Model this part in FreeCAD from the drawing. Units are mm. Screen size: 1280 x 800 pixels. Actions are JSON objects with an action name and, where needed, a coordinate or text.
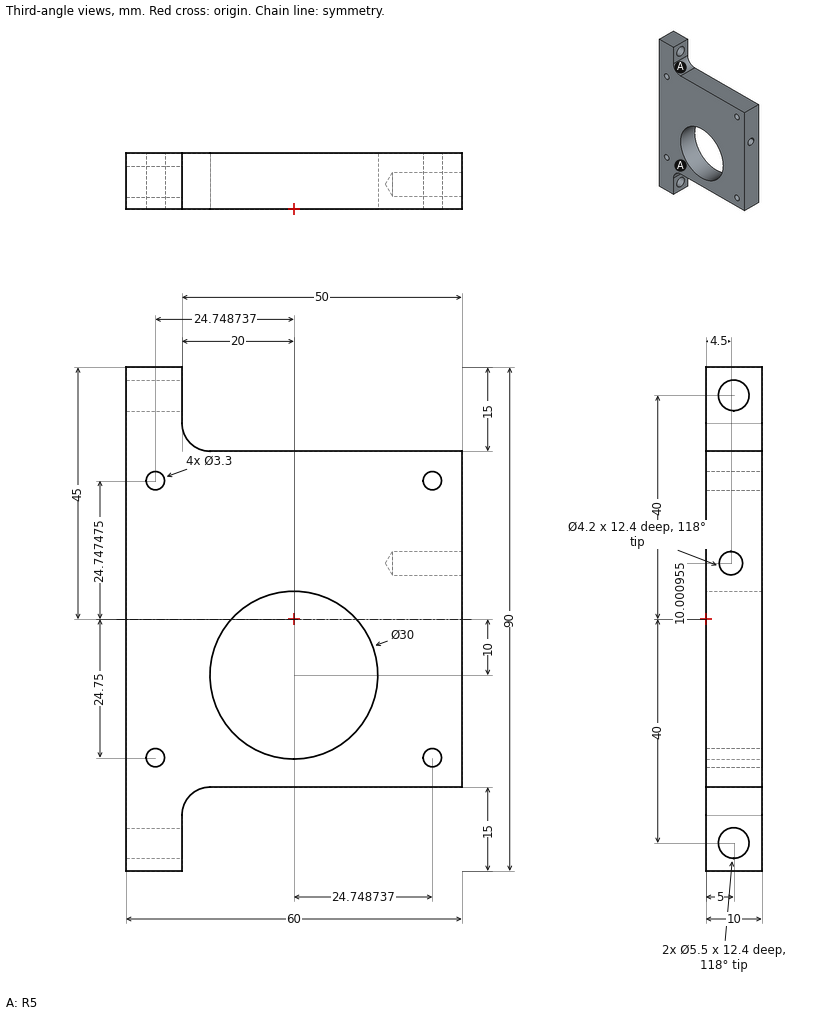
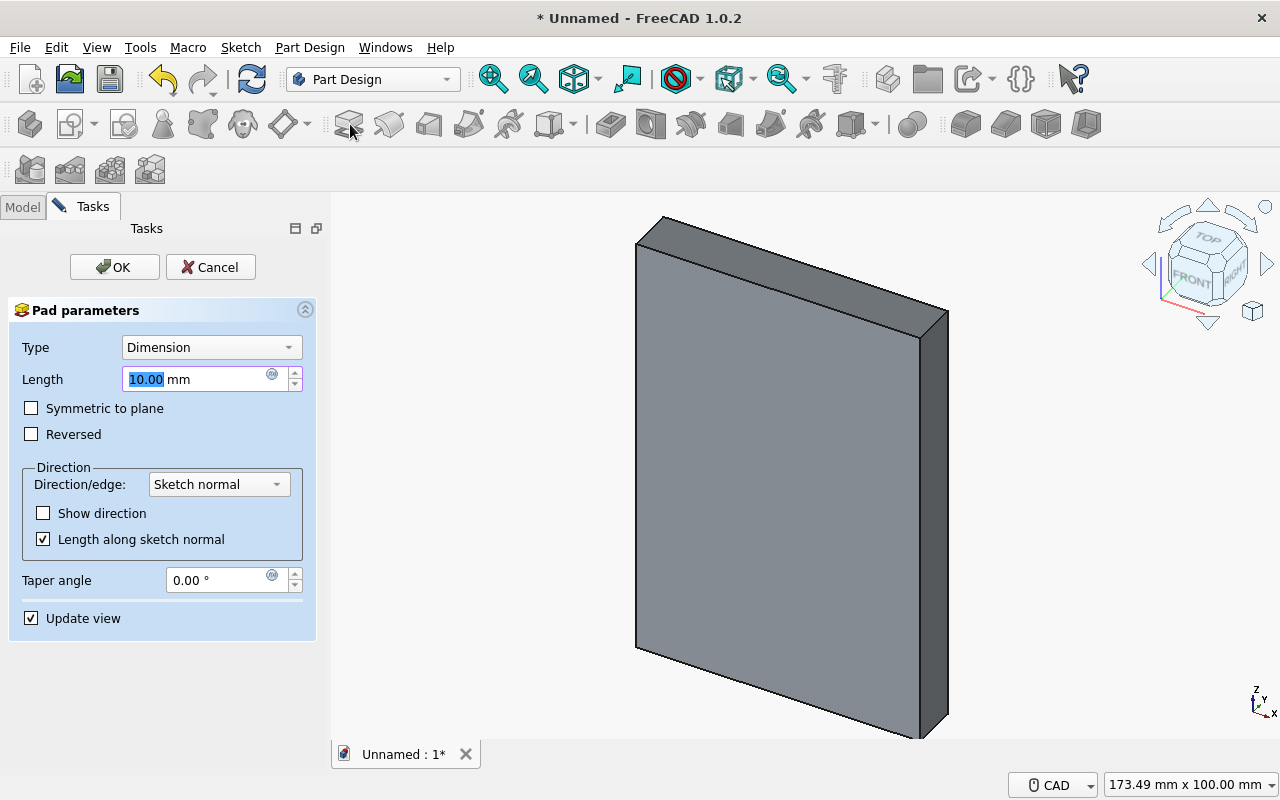
{"action": "type", "text": "10"}
{"action": "key", "text": "Tab"}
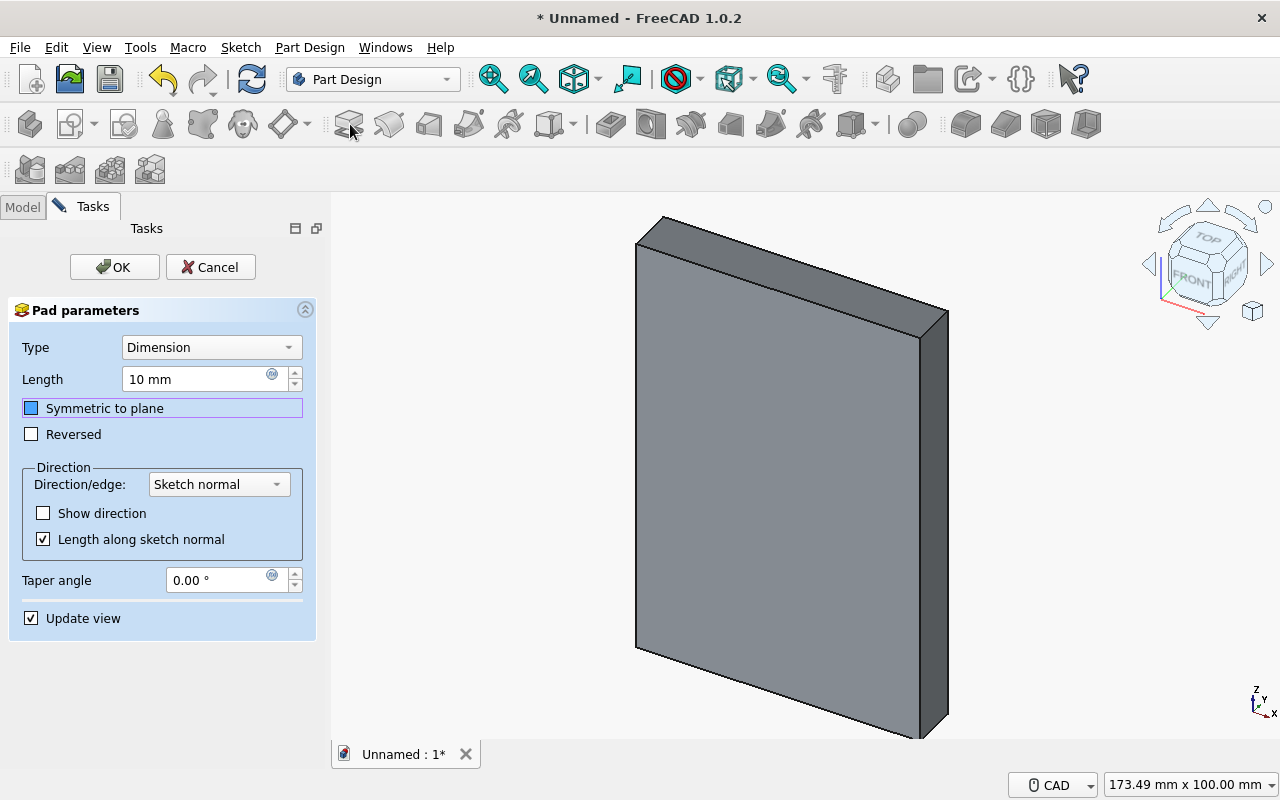
{"action": "left_click", "coordinate": [30, 434]}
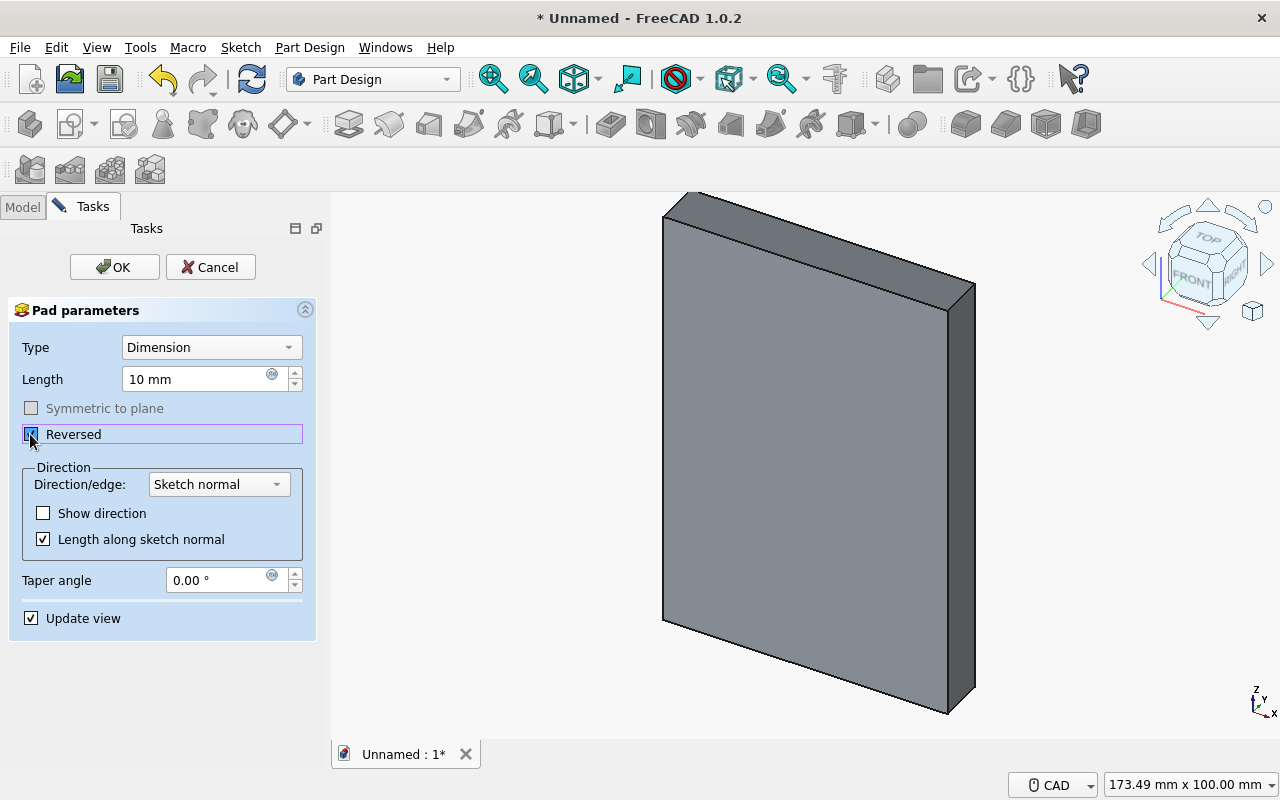
{"action": "left_click", "coordinate": [115, 267]}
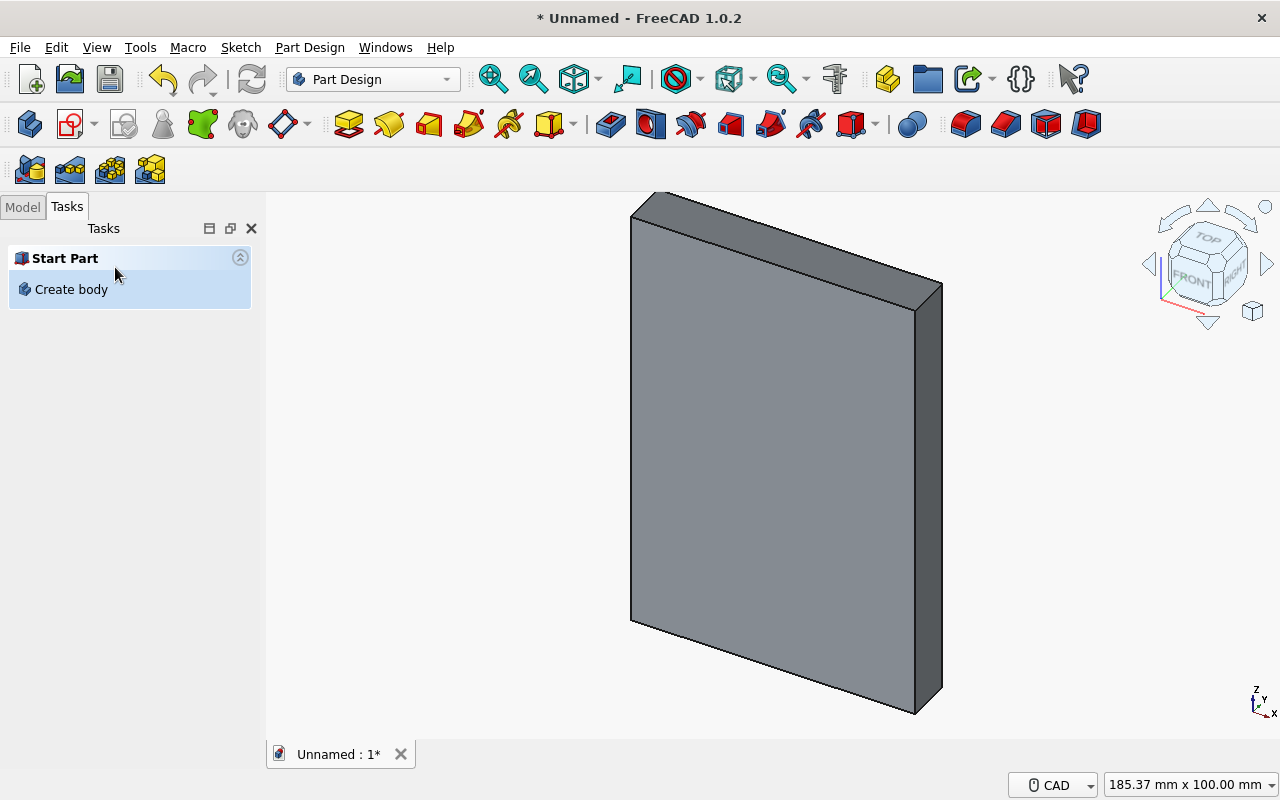
{"action": "key", "text": "v f"}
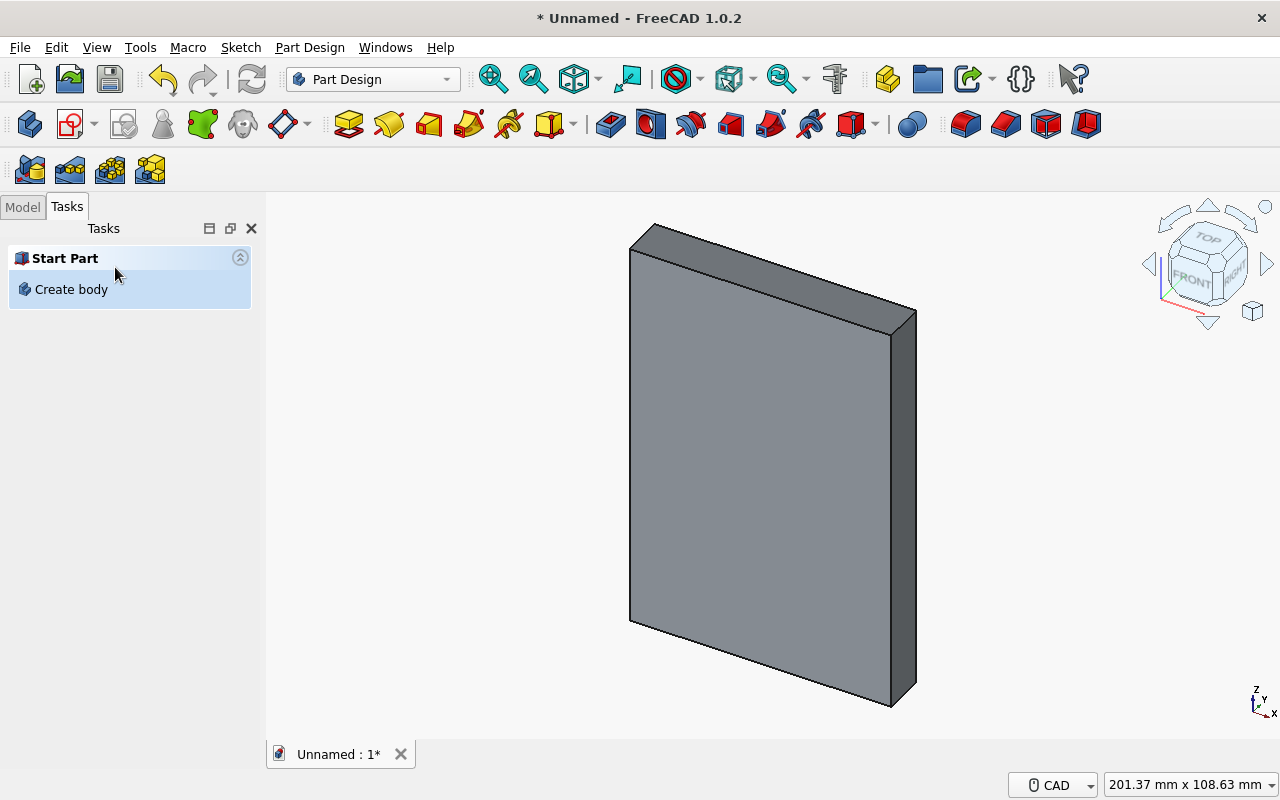
{"action": "left_click", "coordinate": [760, 424]}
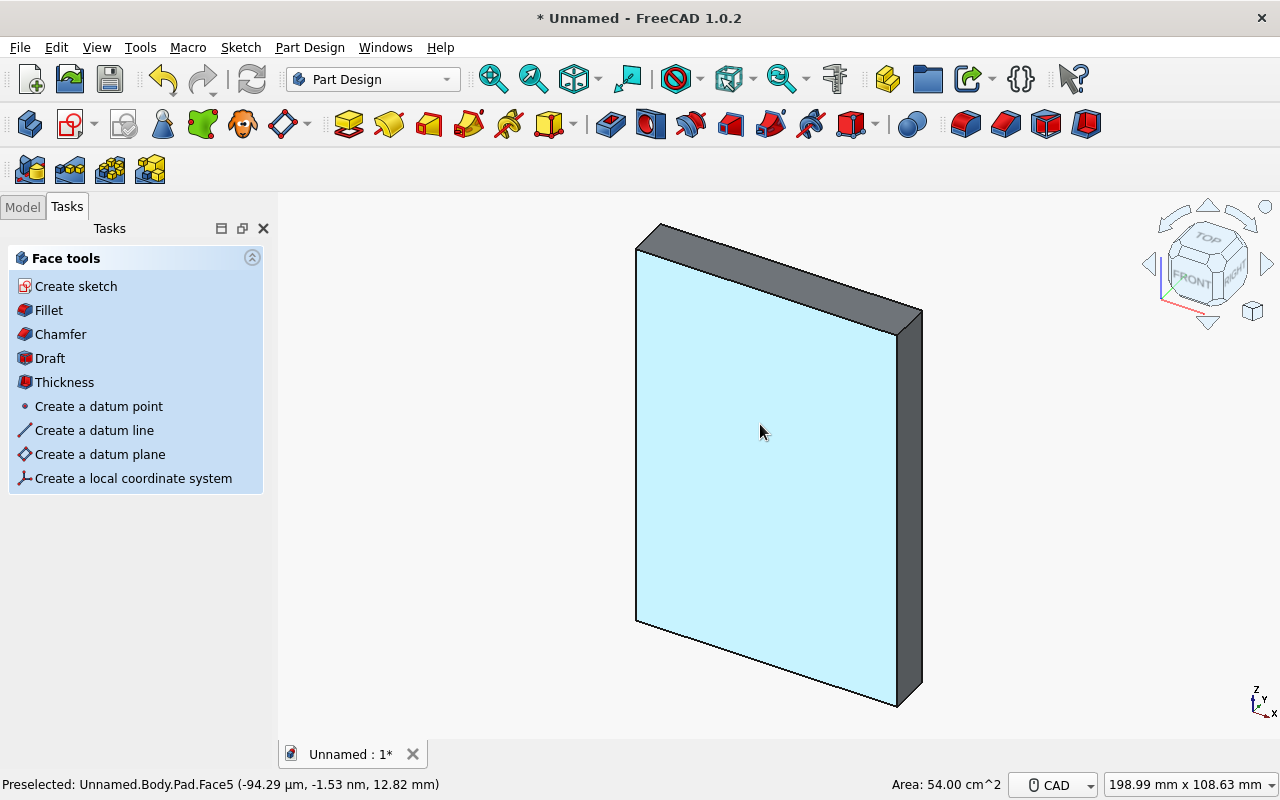
{"action": "left_click", "coordinate": [70, 124]}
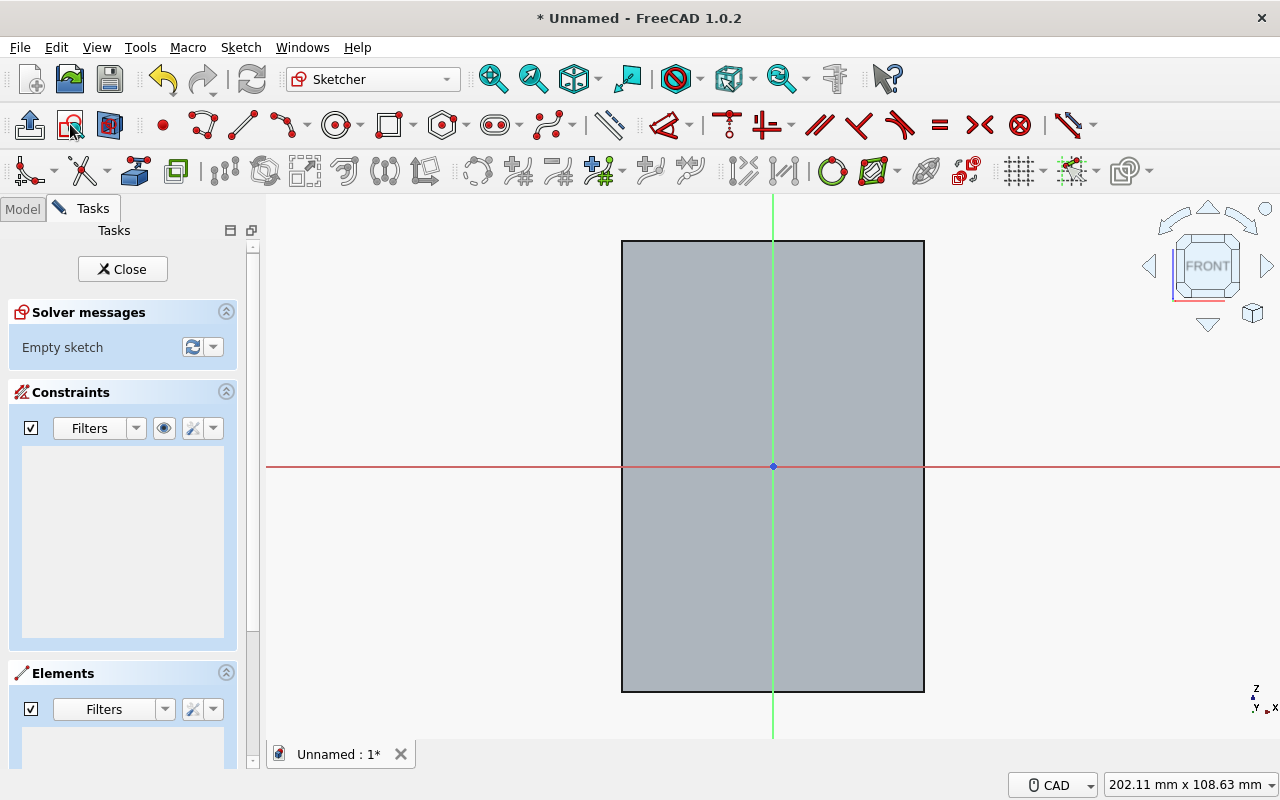
{"action": "scroll", "coordinate": [829, 558], "scroll_direction": "up", "scroll_amount": 4}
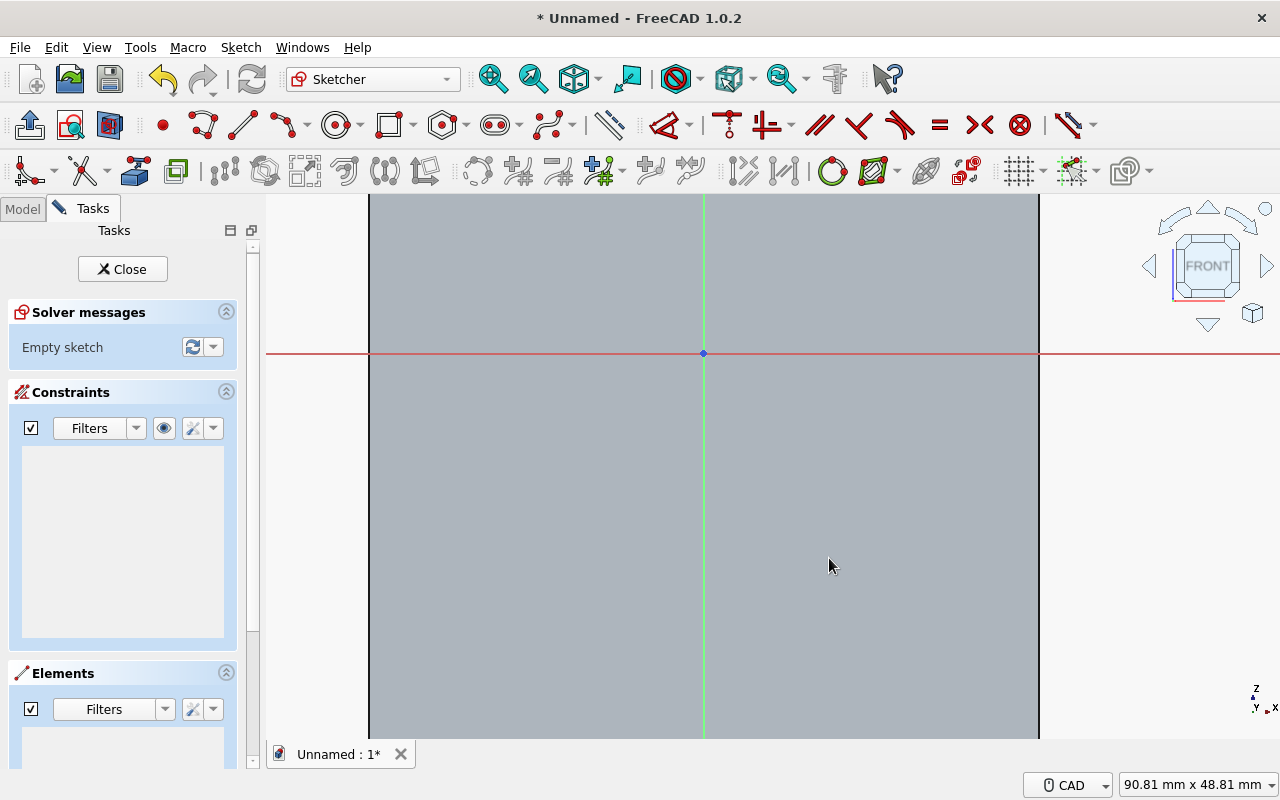
{"action": "key", "text": "g c"}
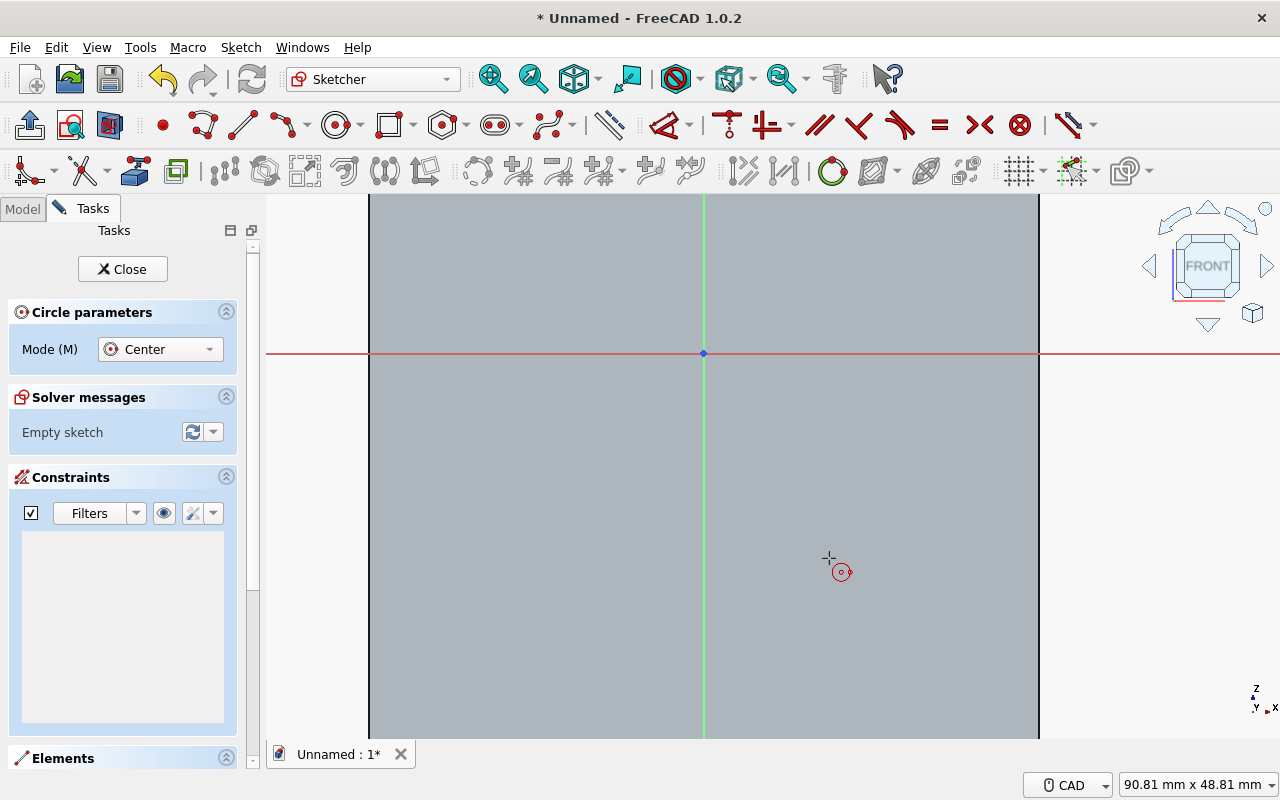
{"action": "left_click", "coordinate": [704, 465]}
{"action": "mouse_move", "coordinate": [822, 584]}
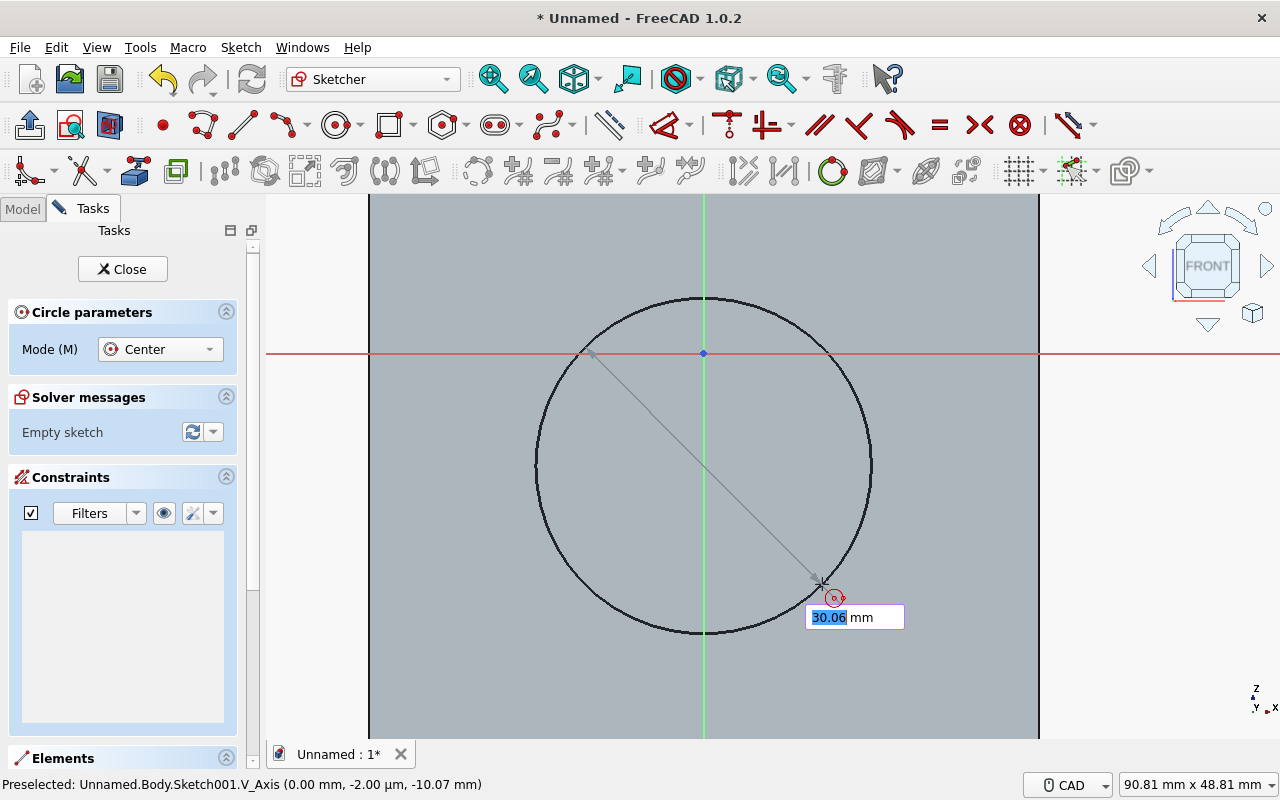
{"action": "type", "text": "30"}
{"action": "key", "text": "Return"}
{"action": "key", "text": "Escape"}